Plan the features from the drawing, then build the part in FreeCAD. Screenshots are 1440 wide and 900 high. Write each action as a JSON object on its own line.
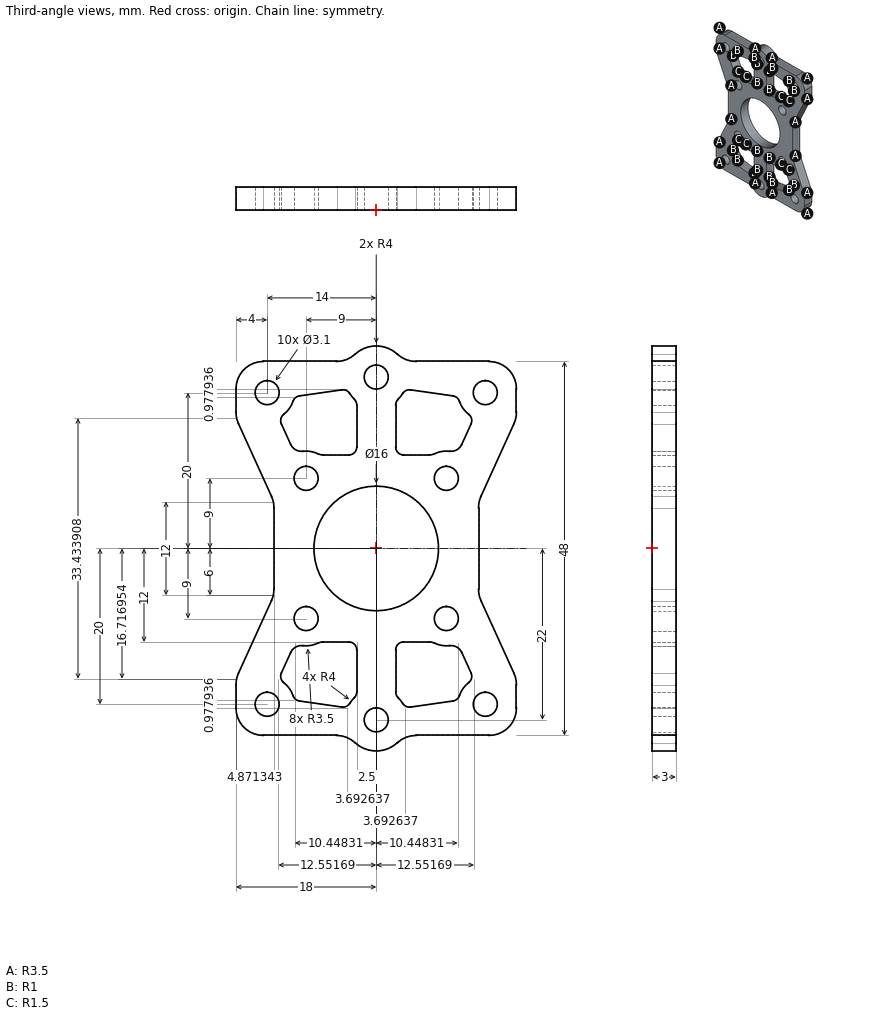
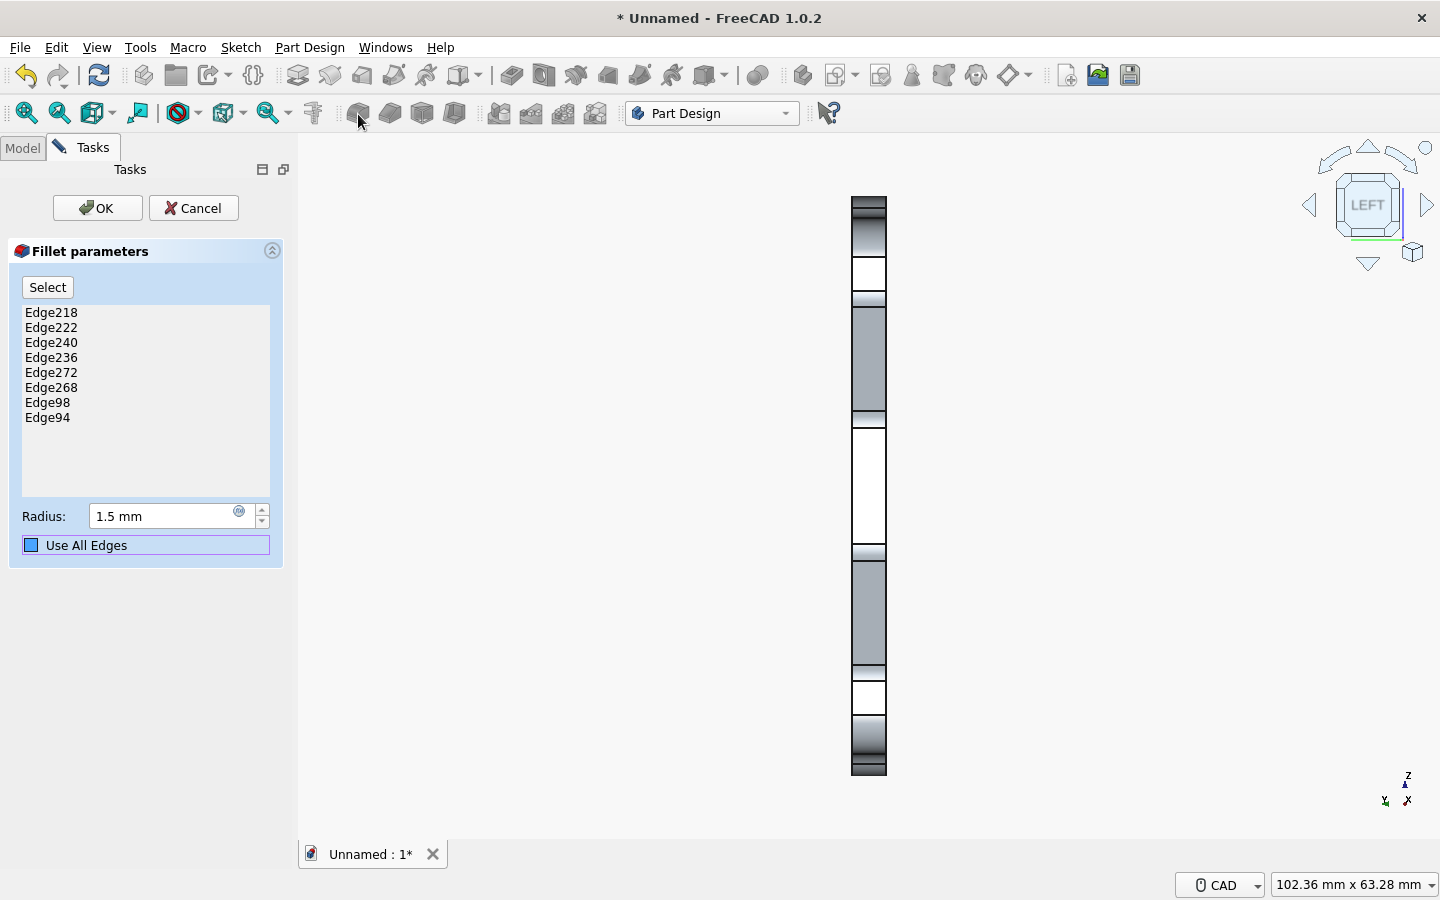
{"action": "left_click", "coordinate": [98, 208]}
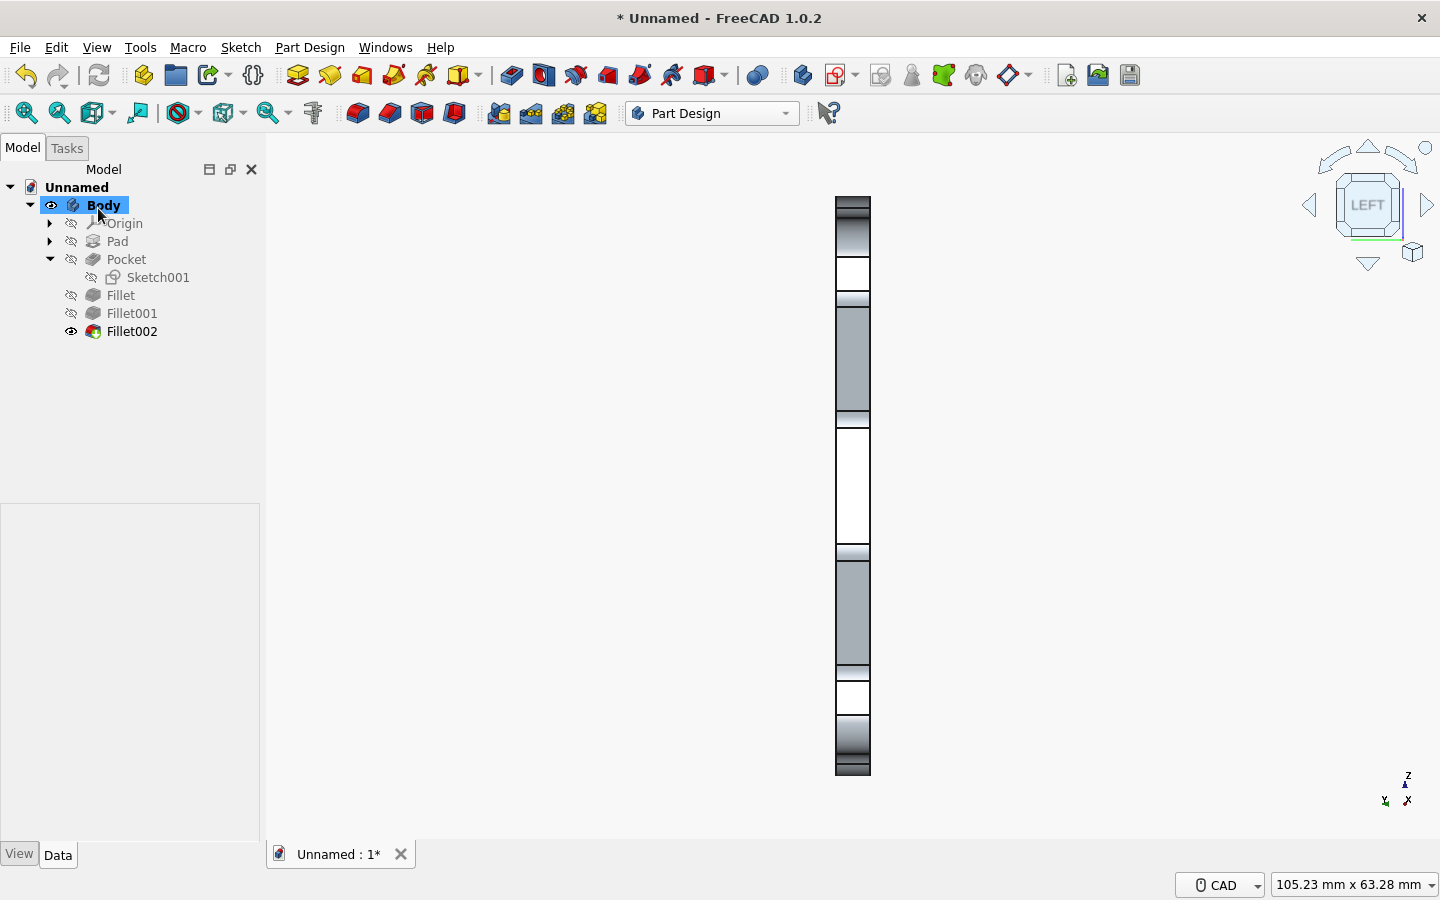
{"action": "key", "text": "0"}